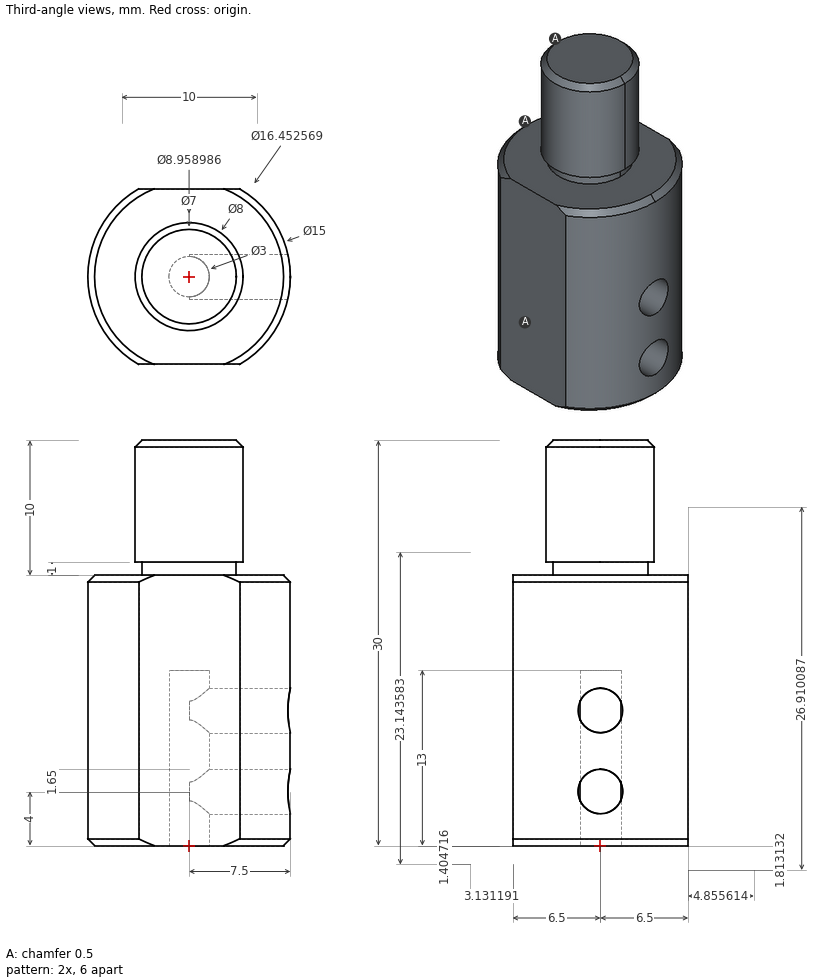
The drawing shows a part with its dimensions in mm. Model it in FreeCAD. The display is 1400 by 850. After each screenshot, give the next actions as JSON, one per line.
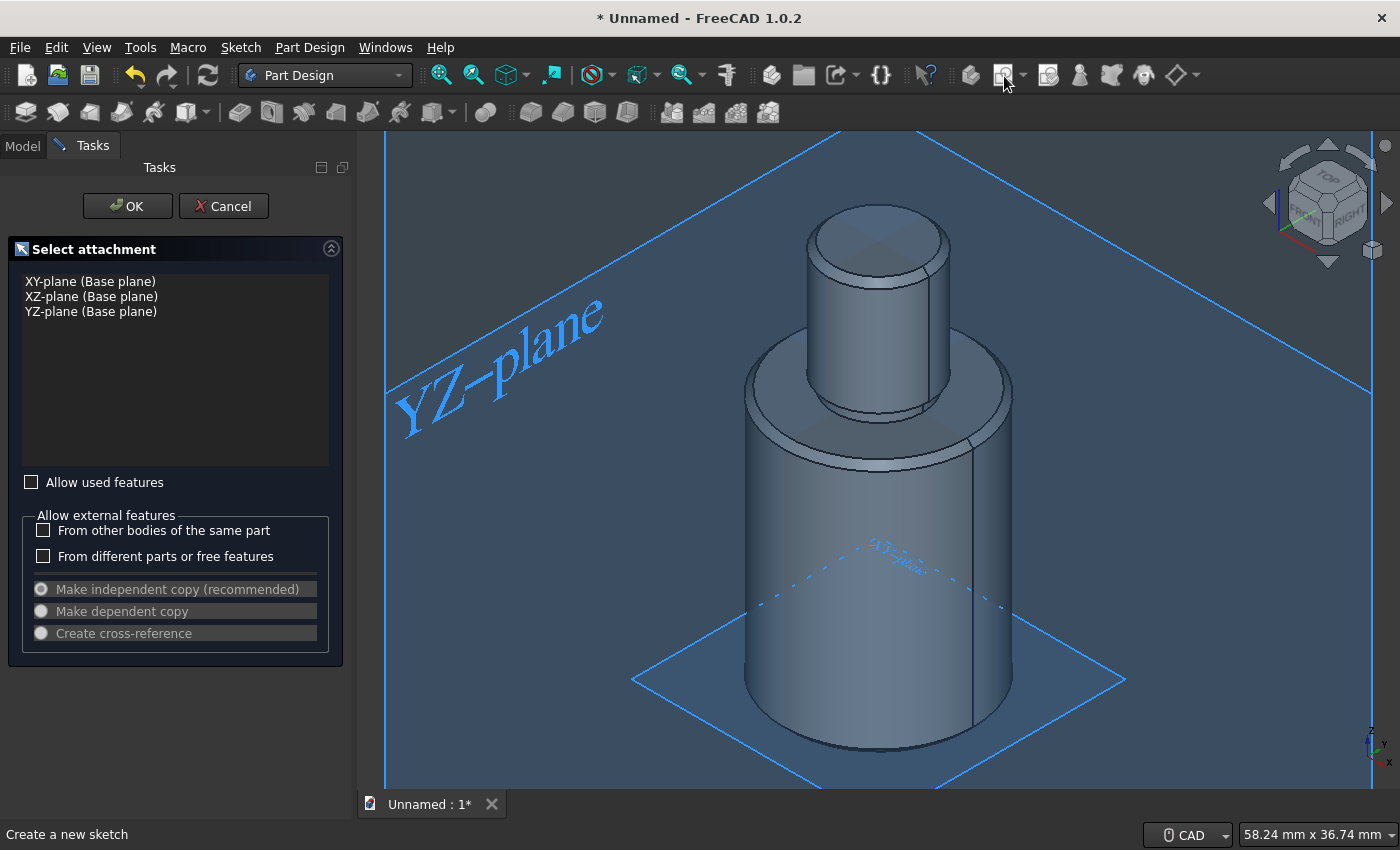
{"action": "left_click", "coordinate": [82, 296]}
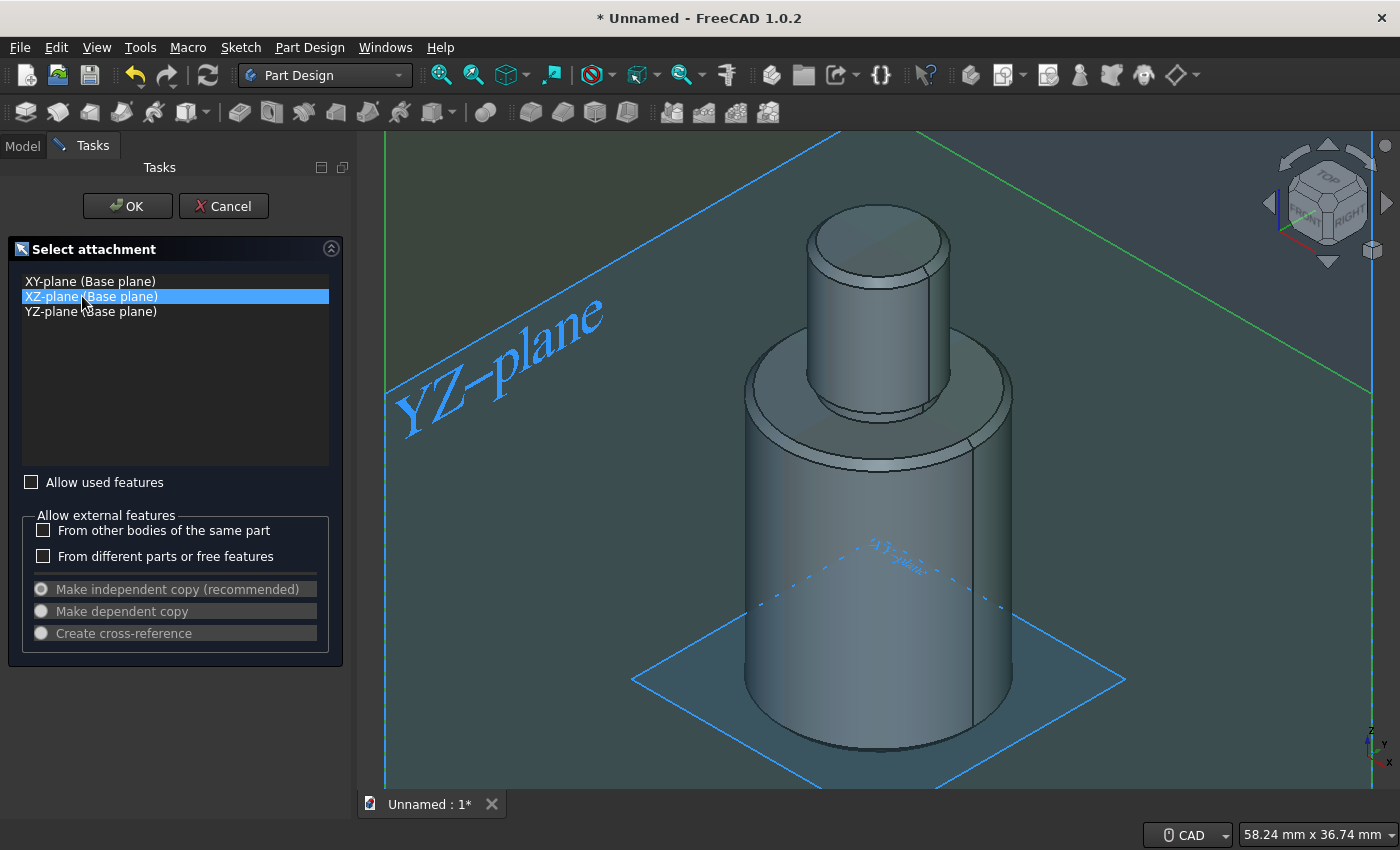
{"action": "left_click", "coordinate": [128, 206]}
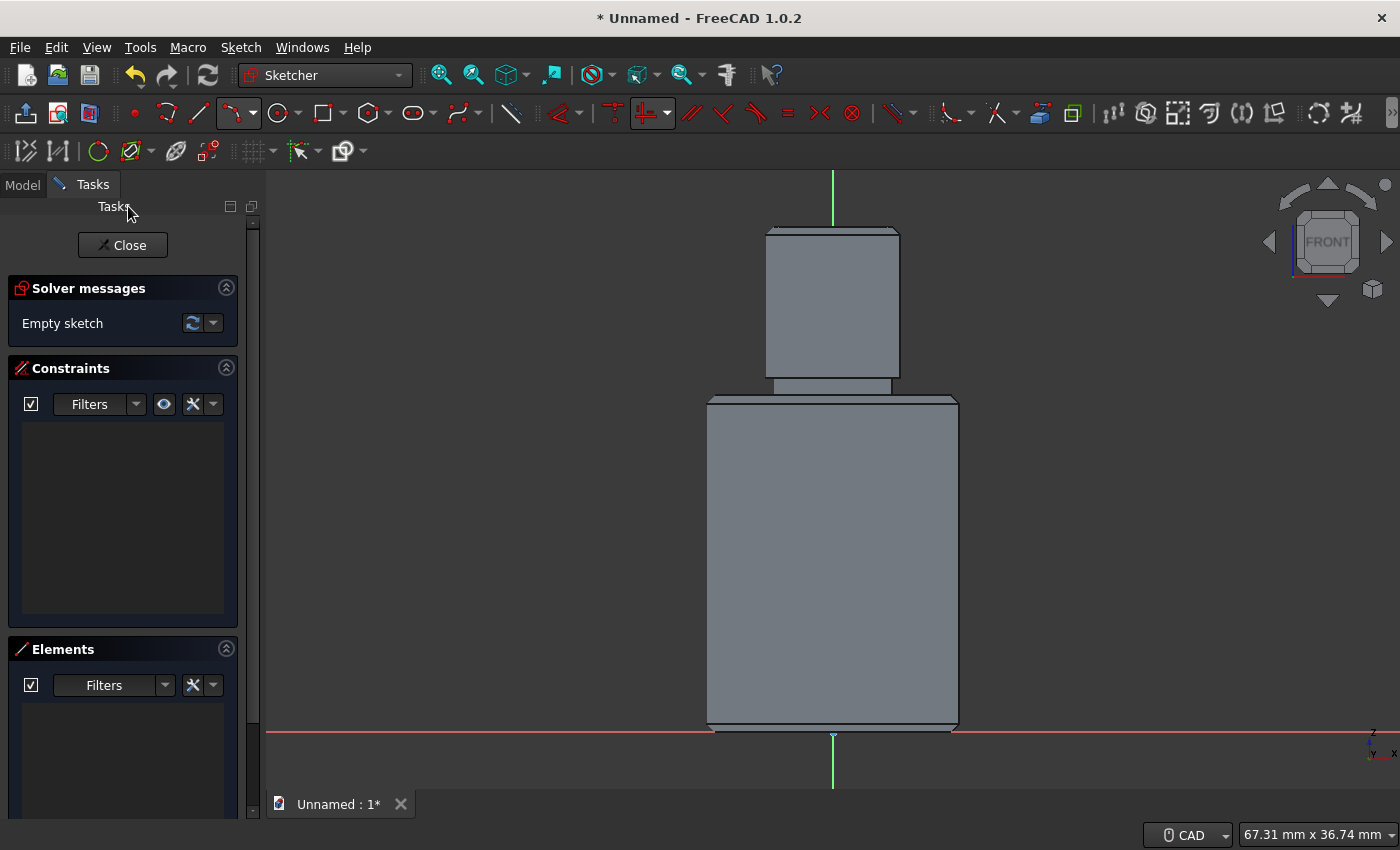
{"action": "left_click", "coordinate": [90, 114]}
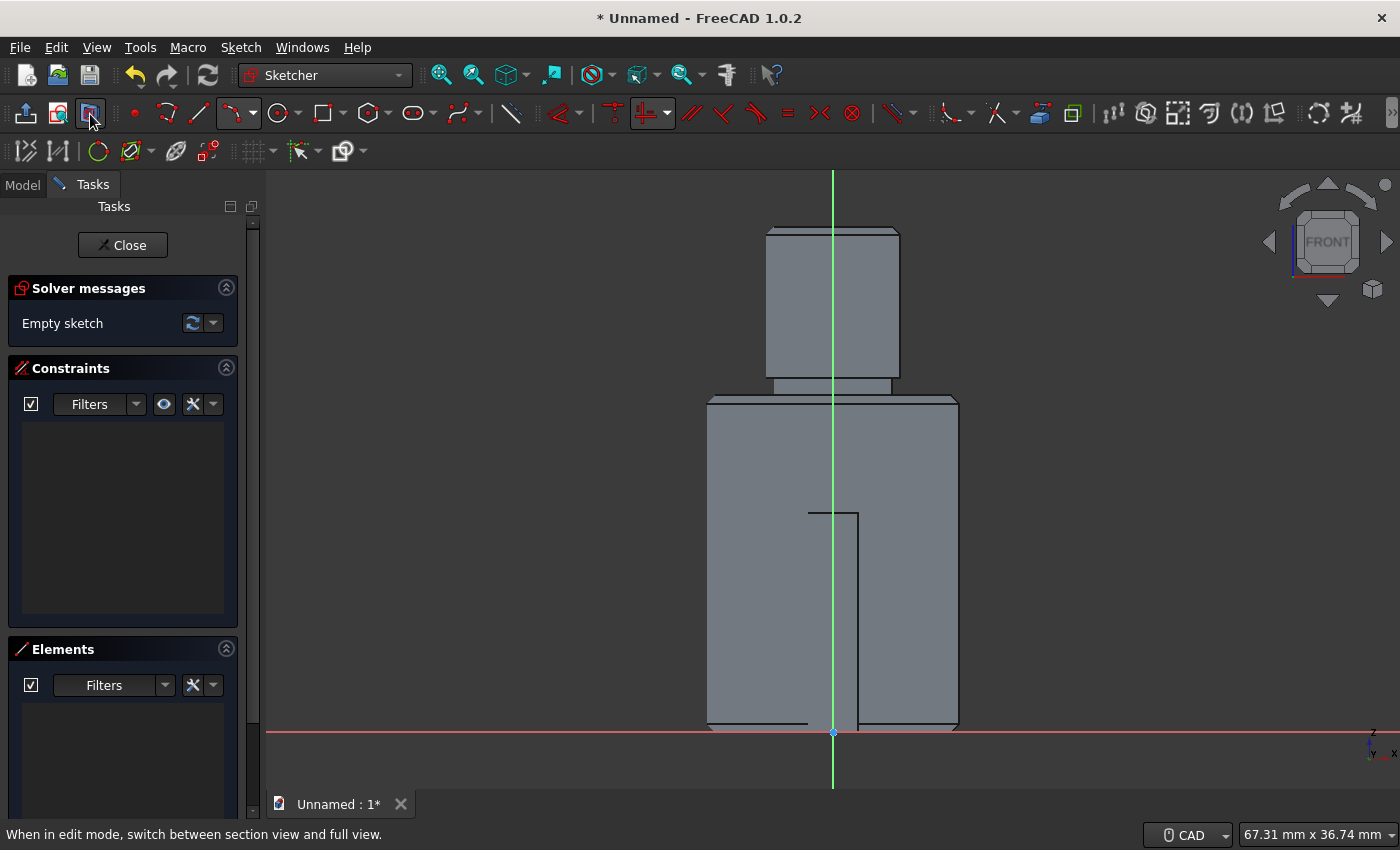
{"action": "scroll", "coordinate": [973, 752], "scroll_direction": "up", "scroll_amount": 7}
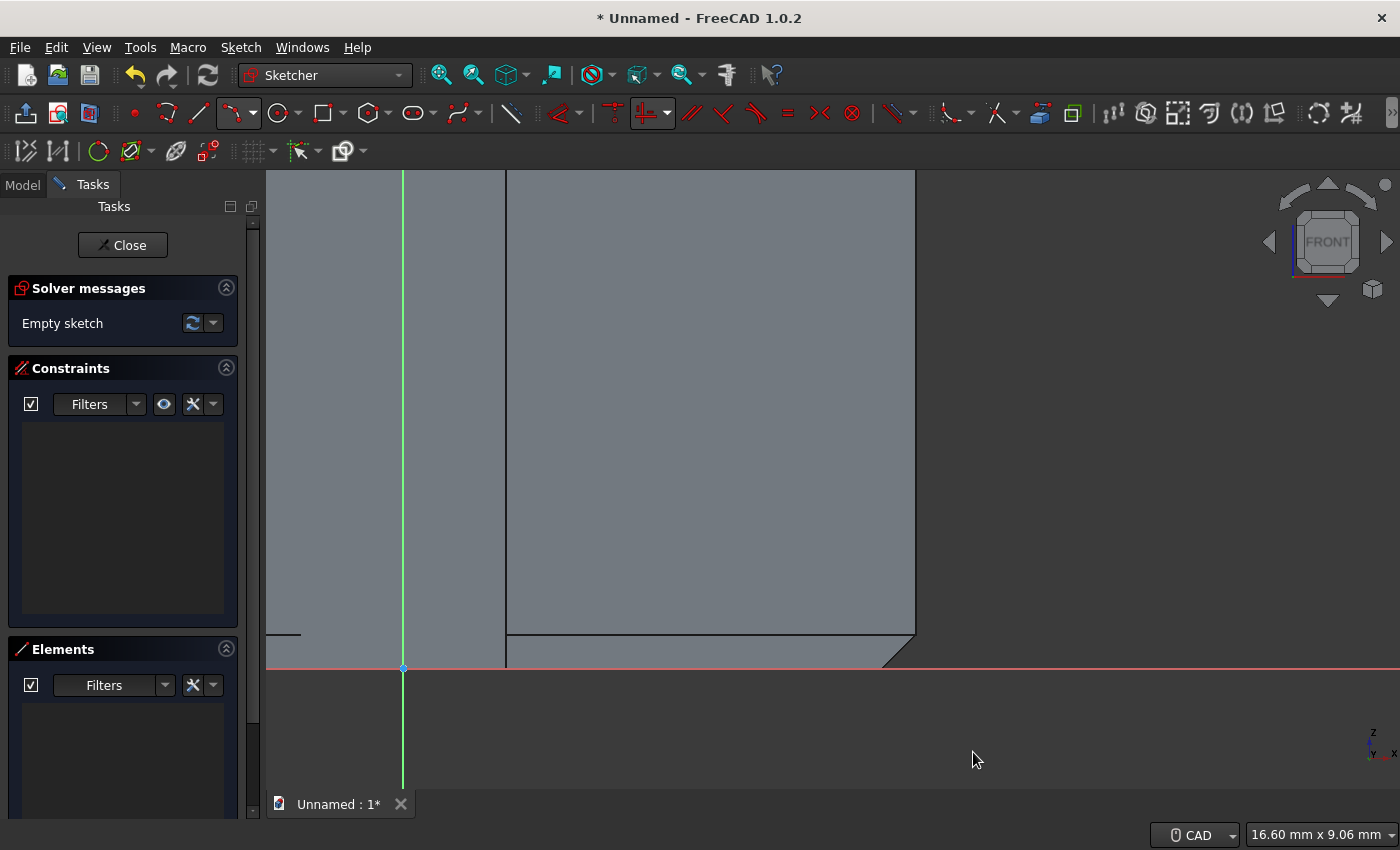
{"action": "left_click", "coordinate": [324, 114]}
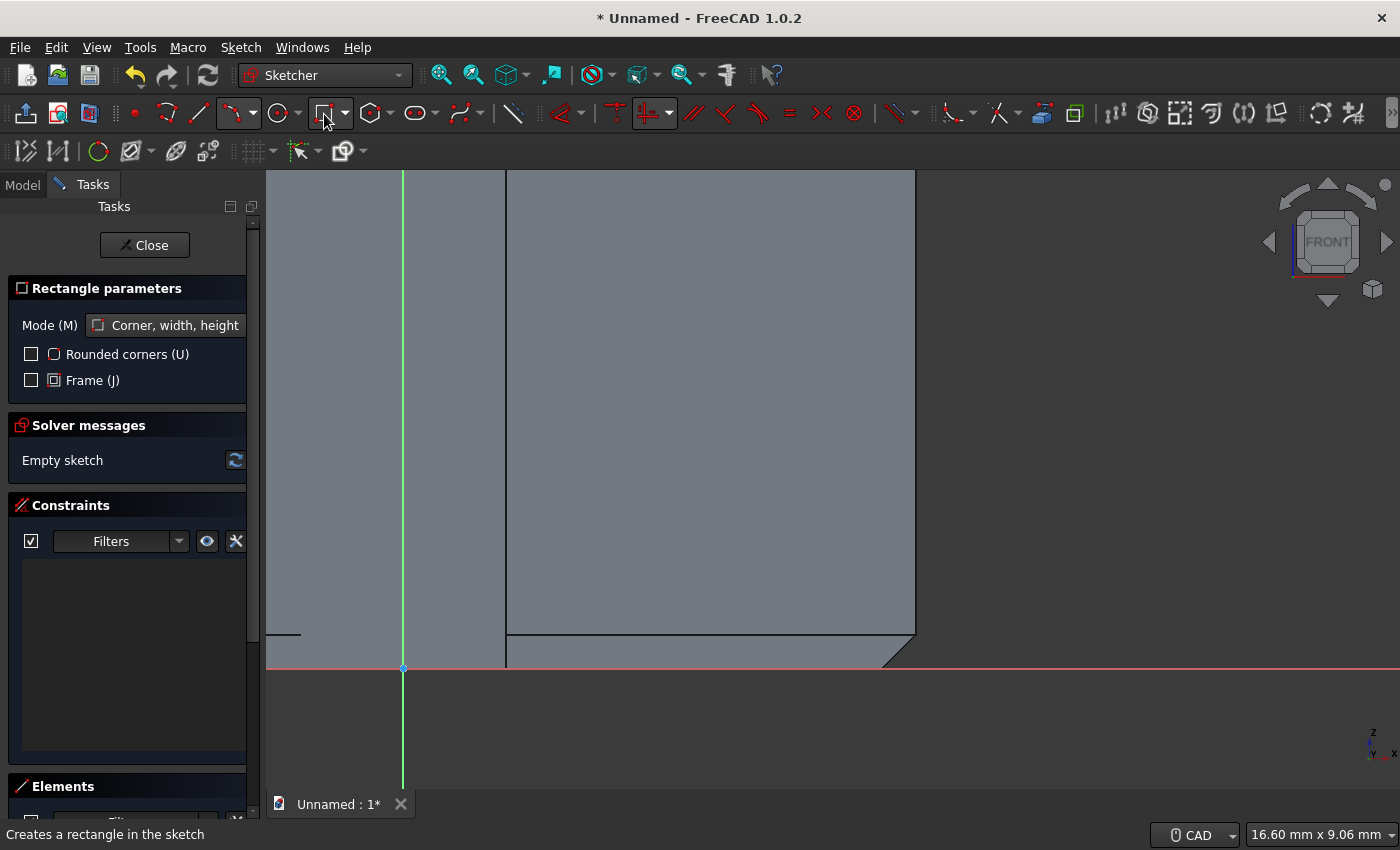
{"action": "left_click", "coordinate": [403, 283]}
{"action": "left_click", "coordinate": [916, 396]}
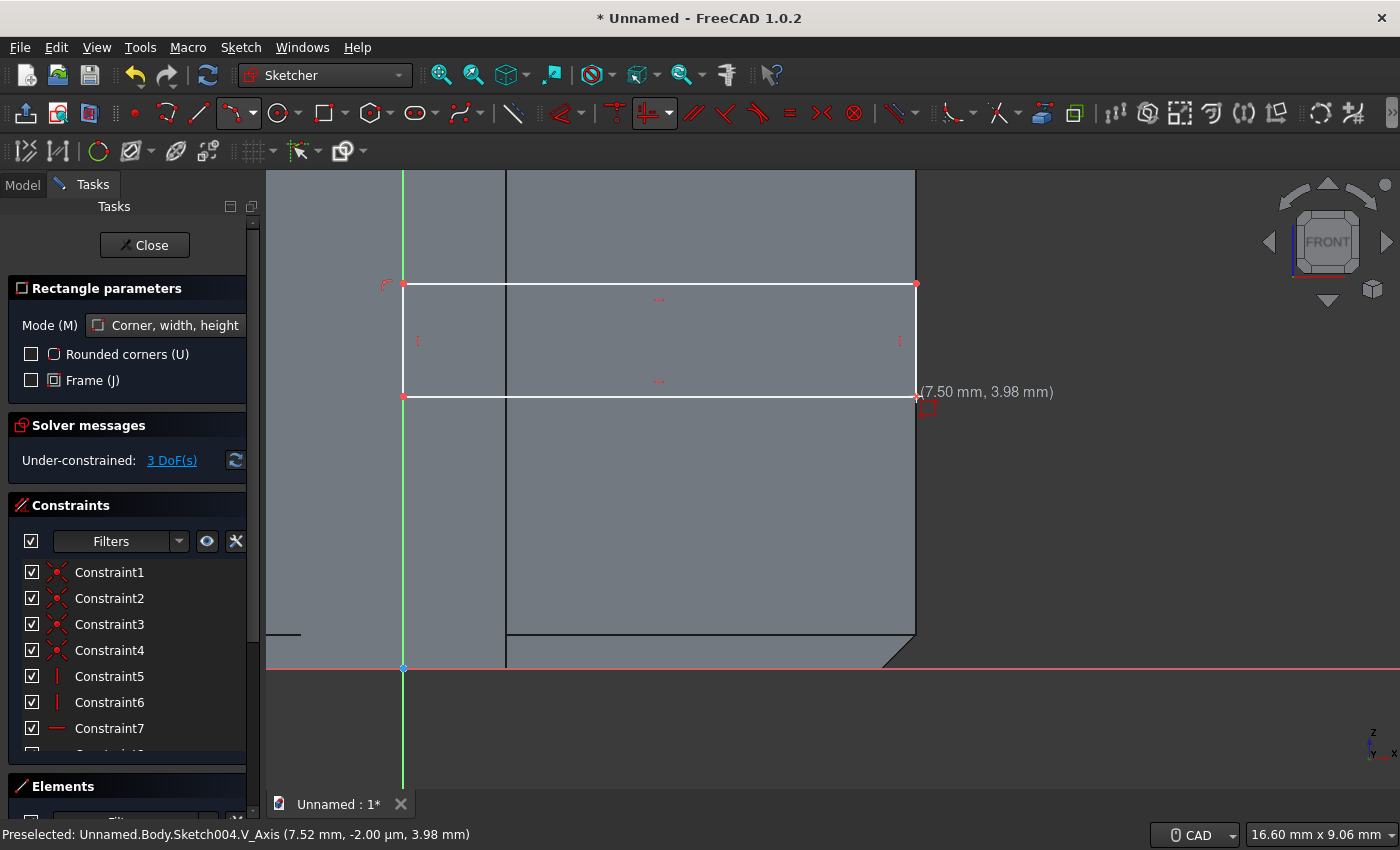
{"action": "left_click", "coordinate": [200, 114]}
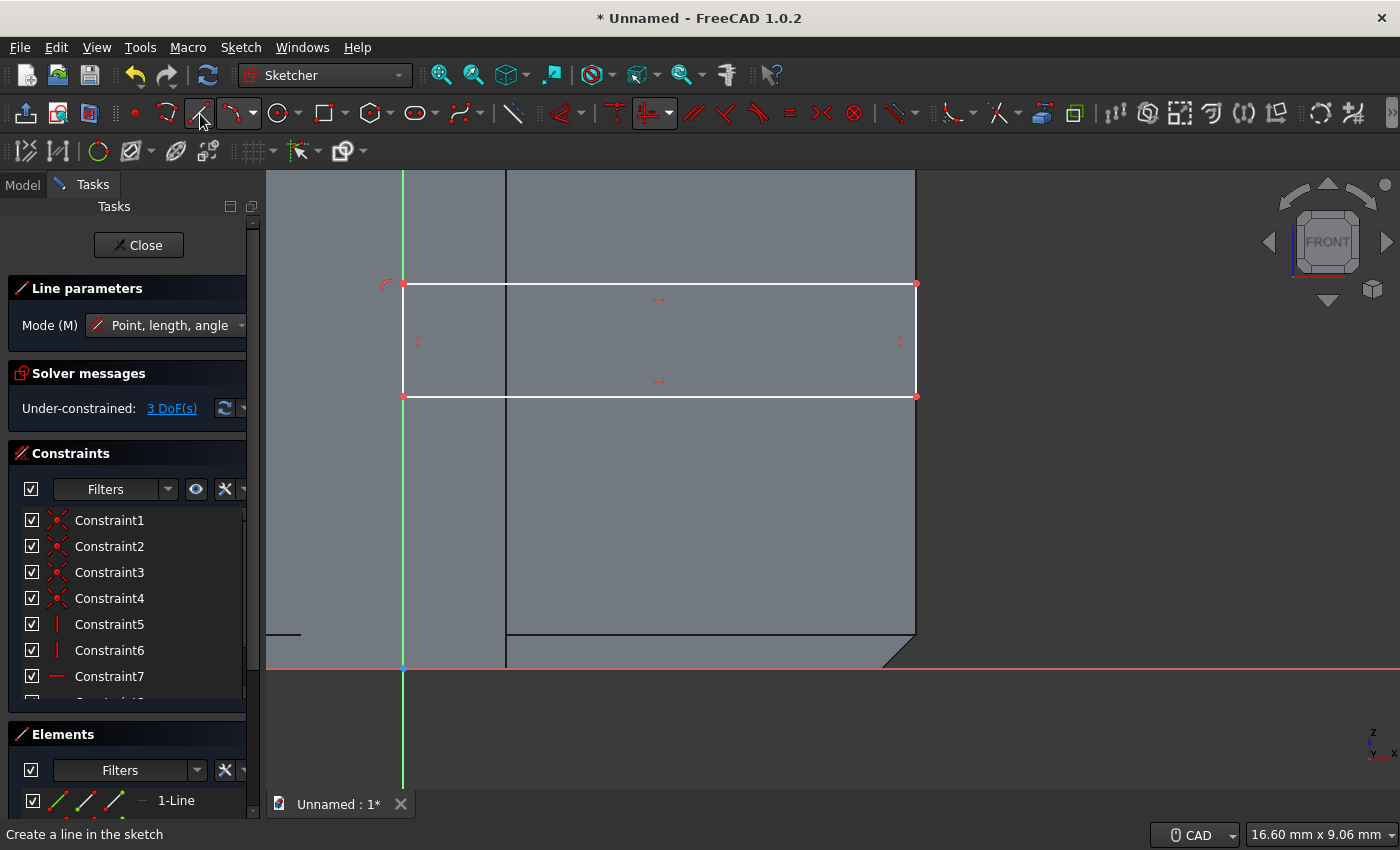
{"action": "left_click", "coordinate": [967, 396]}
{"action": "left_click", "coordinate": [1121, 396]}
{"action": "key", "text": "Escape"}